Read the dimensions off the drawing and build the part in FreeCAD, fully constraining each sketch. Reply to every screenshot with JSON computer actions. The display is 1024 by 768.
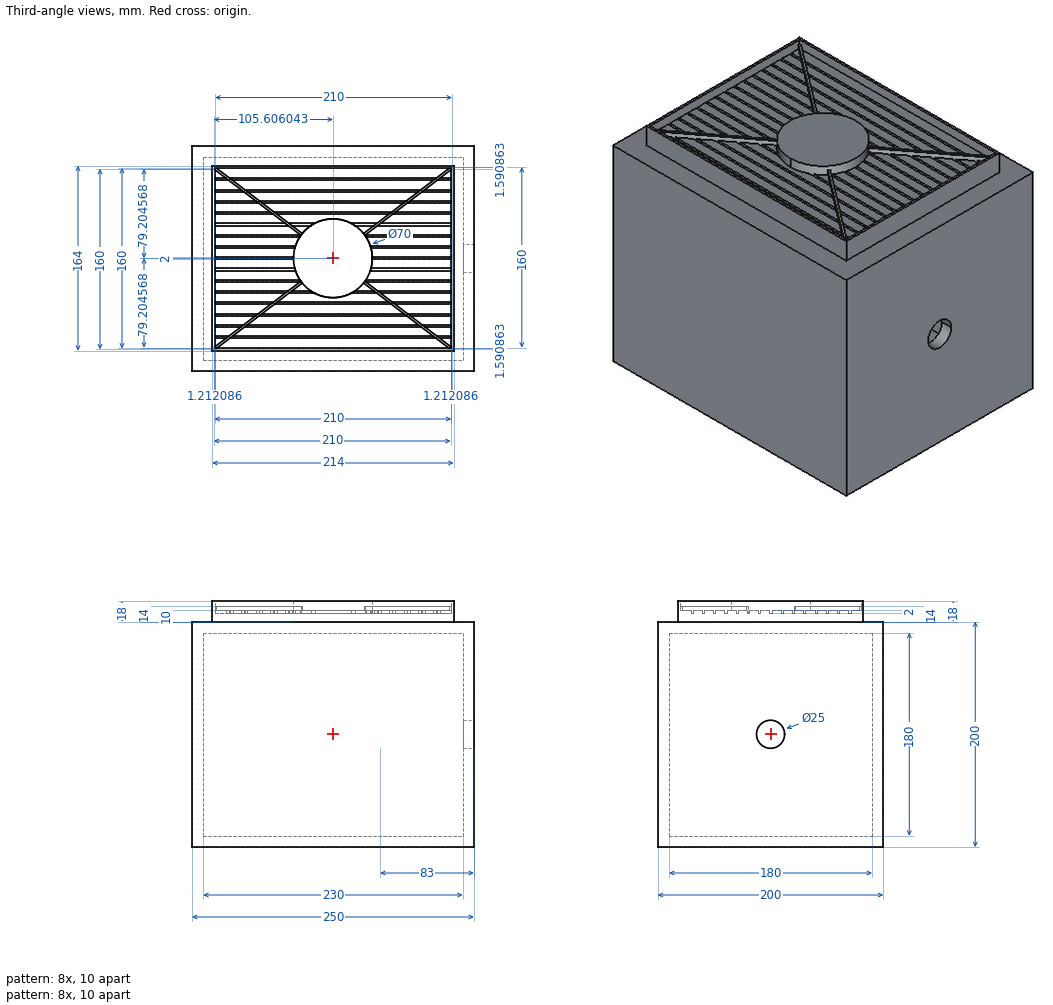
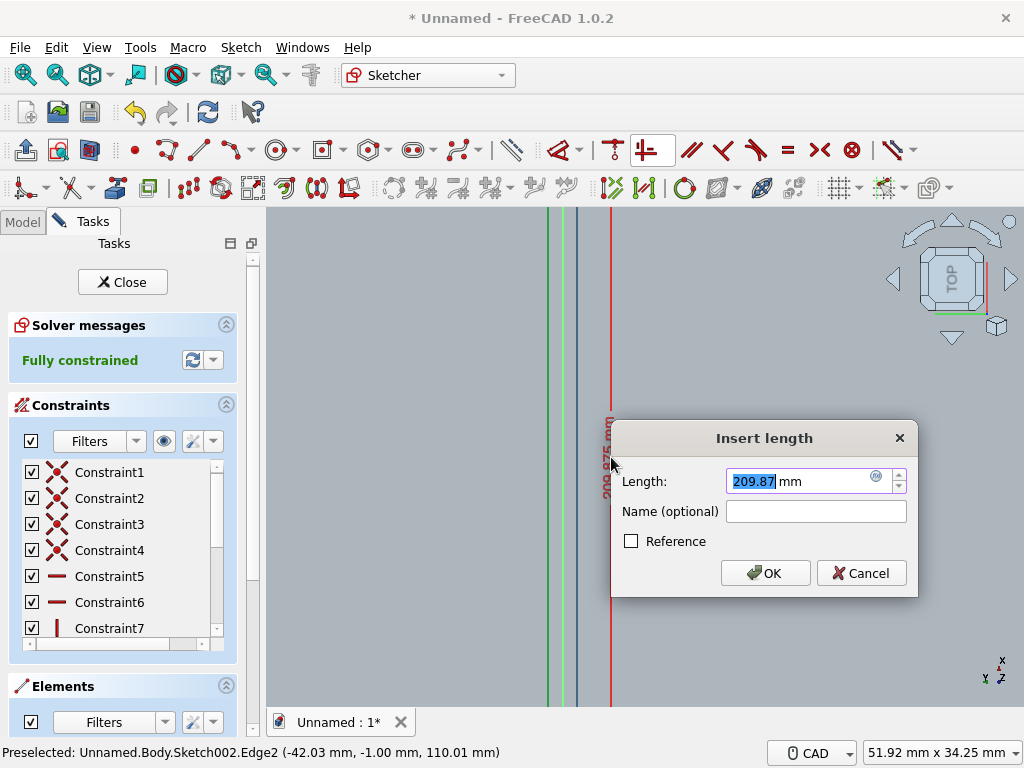
{"action": "type", "text": "210"}
{"action": "key", "text": "Return"}
{"action": "key", "text": "Escape"}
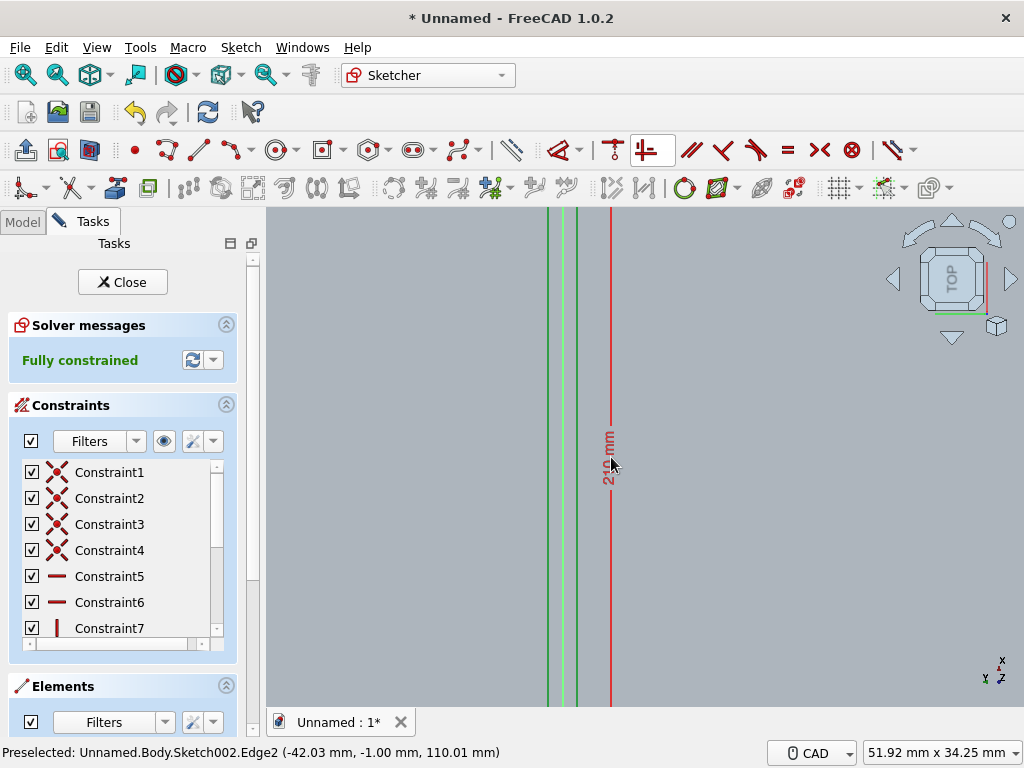
{"action": "left_click", "coordinate": [123, 282]}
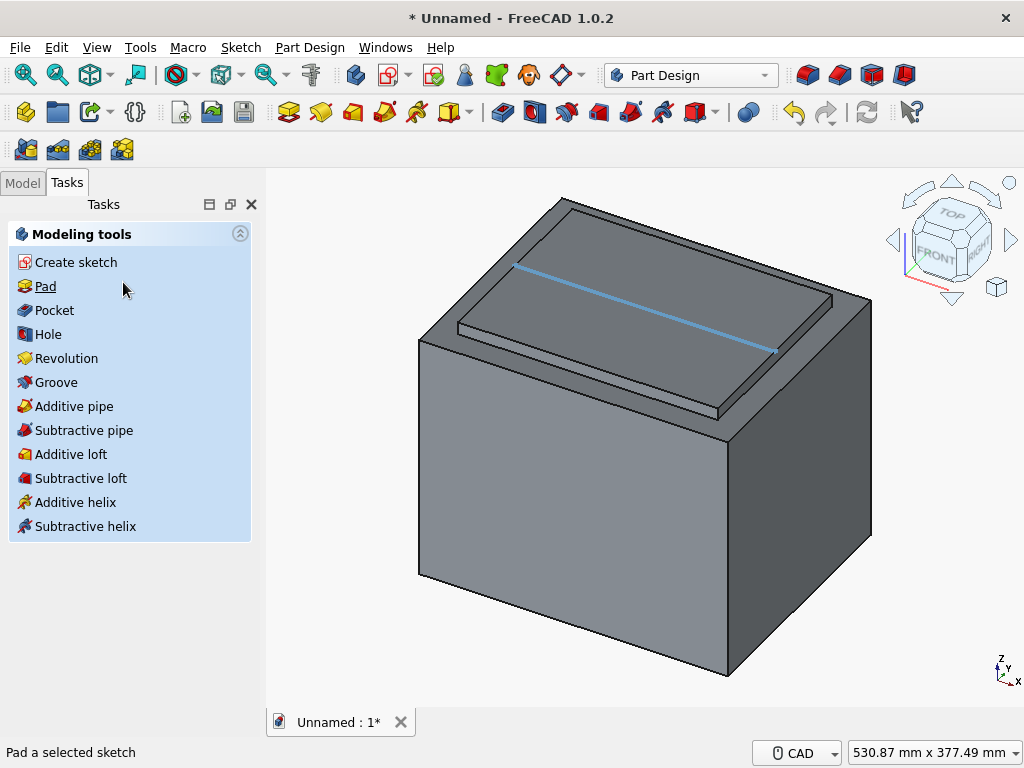
{"action": "left_click", "coordinate": [504, 112]}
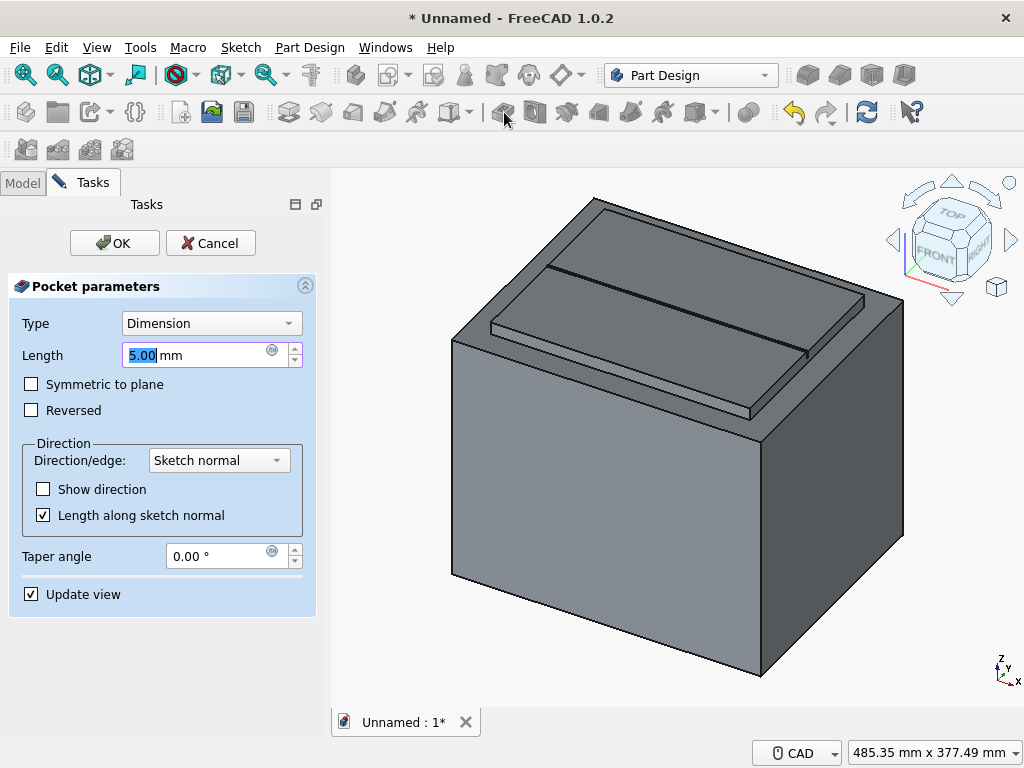
{"action": "type", "text": "2"}
{"action": "key", "text": "Tab"}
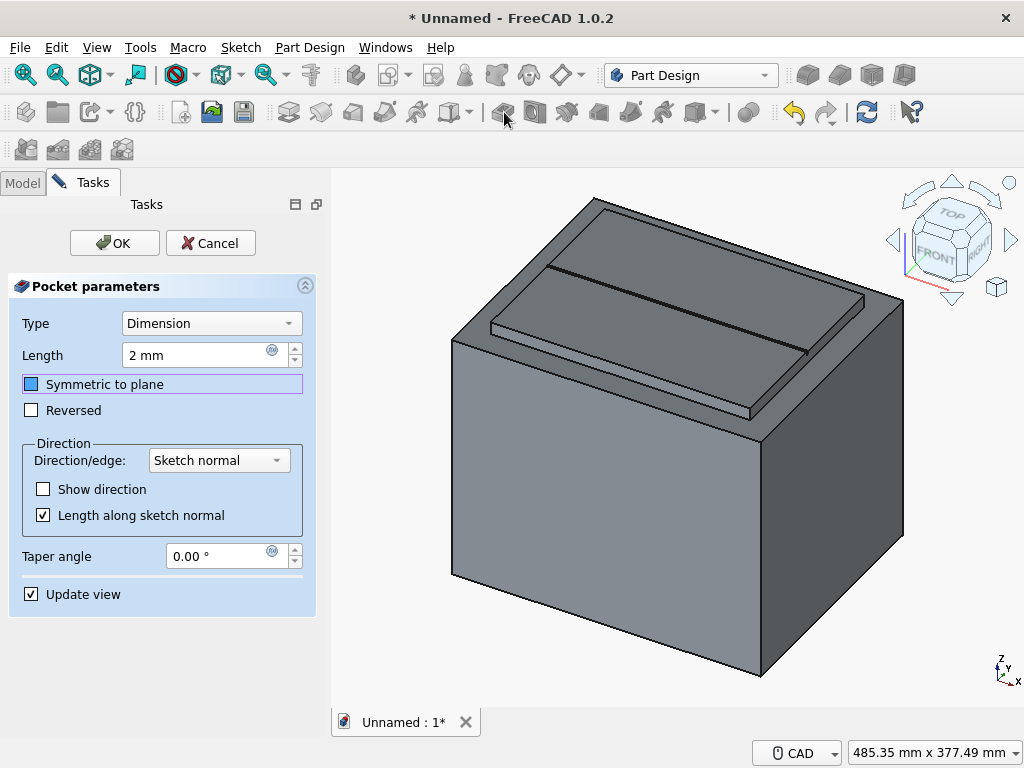
{"action": "left_click", "coordinate": [115, 243]}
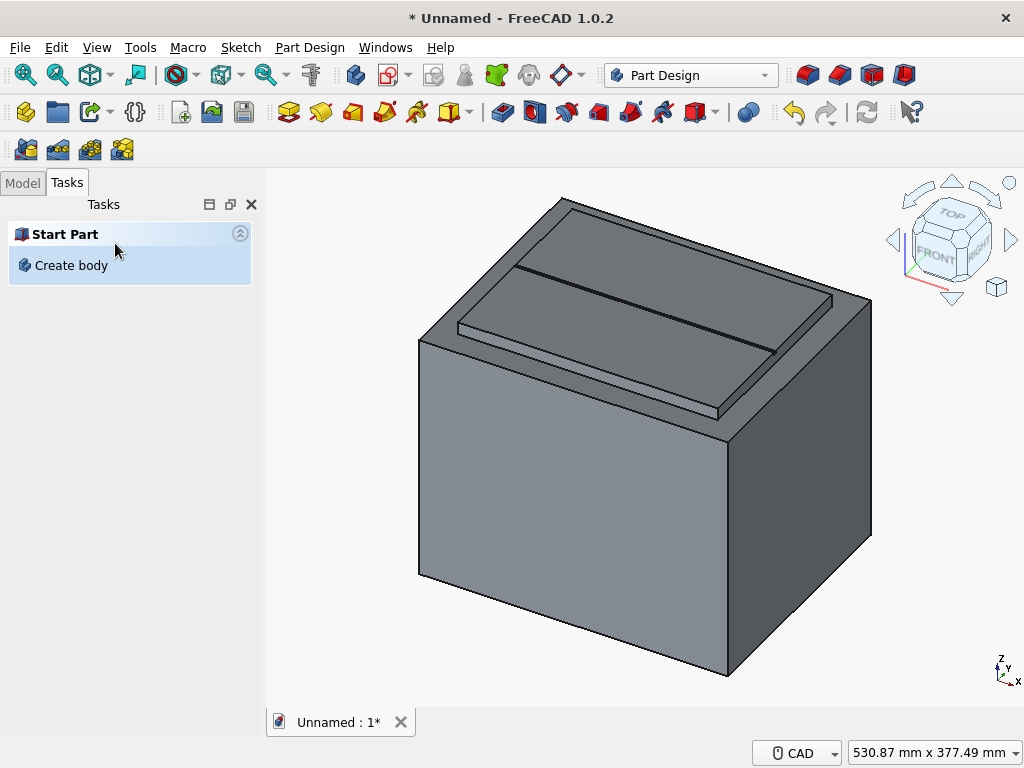
{"action": "left_click", "coordinate": [23, 182]}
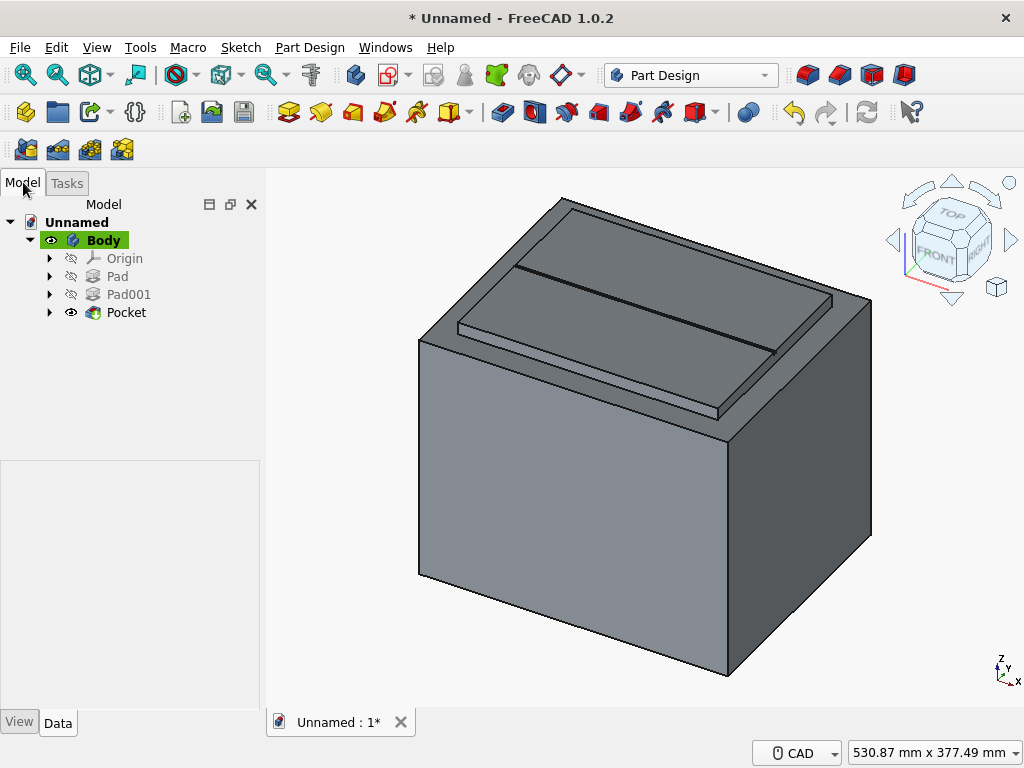
{"action": "left_click", "coordinate": [116, 312]}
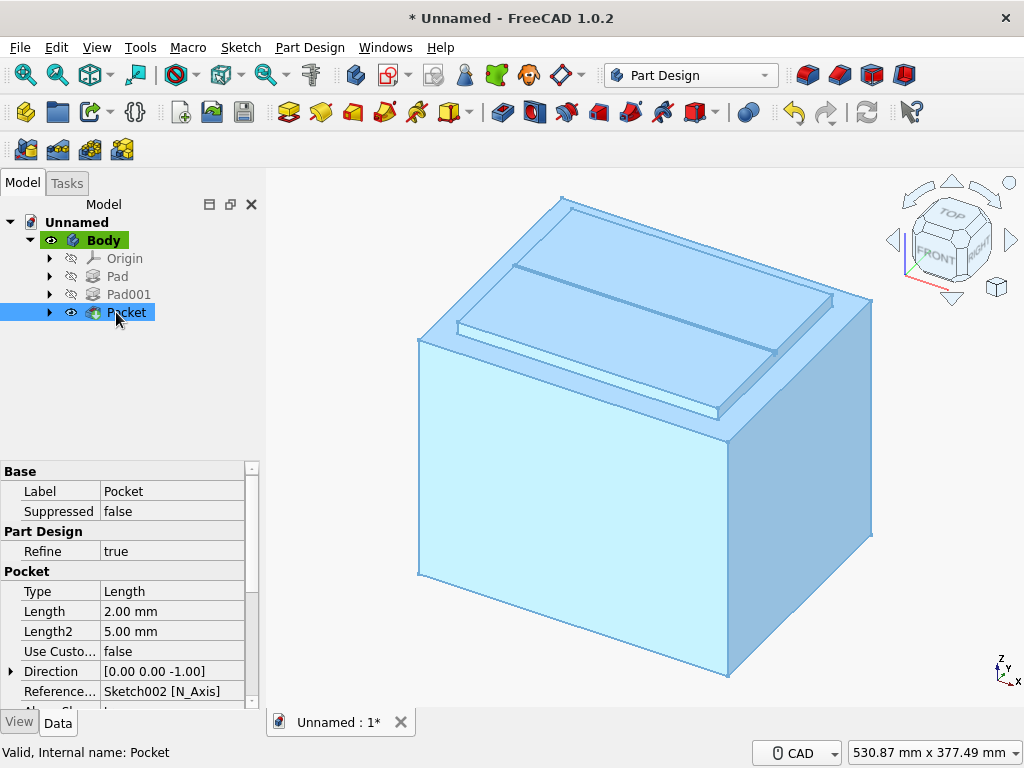
{"action": "left_click", "coordinate": [58, 150]}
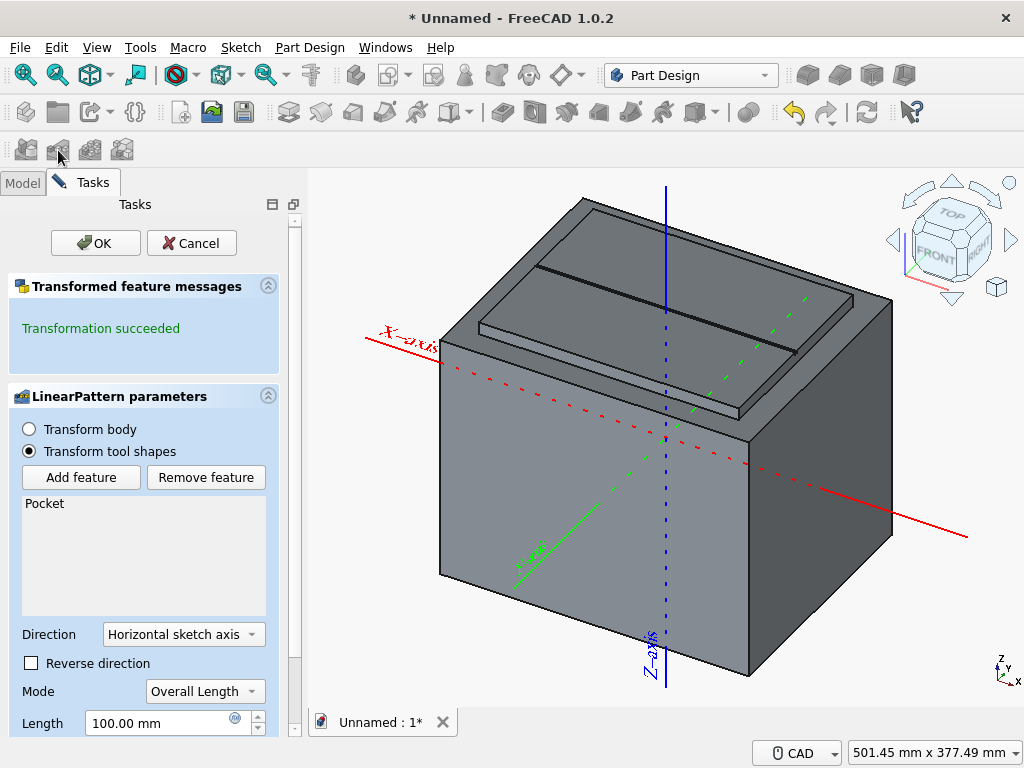
{"action": "left_click", "coordinate": [184, 634]}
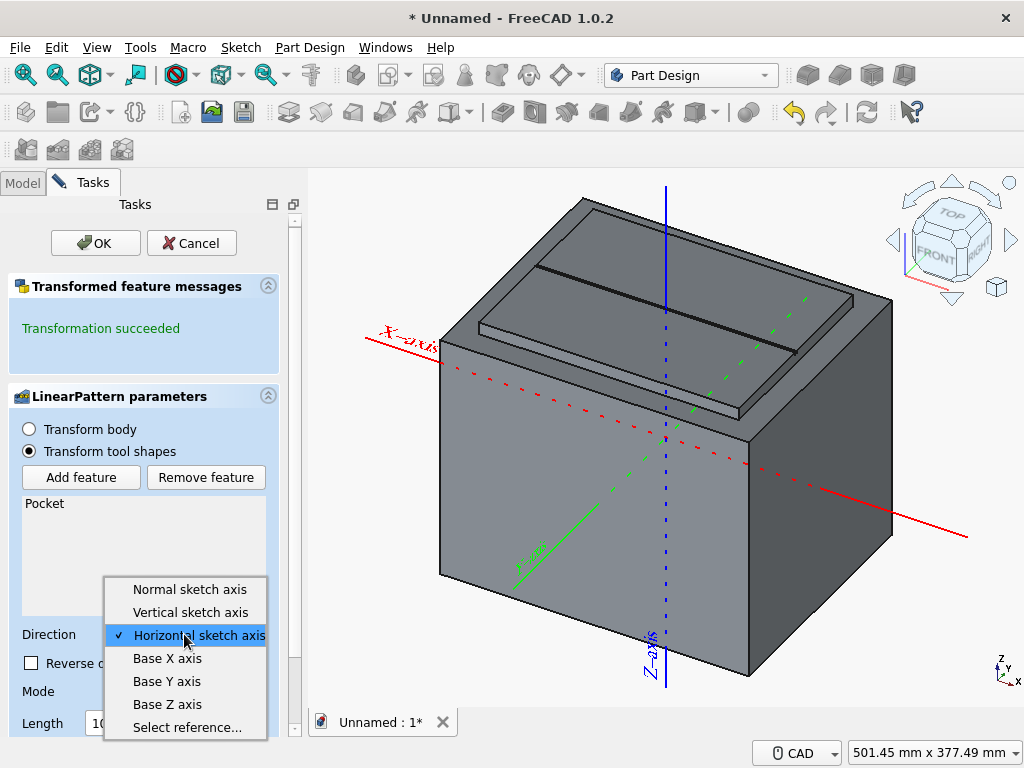
{"action": "left_click", "coordinate": [184, 682]}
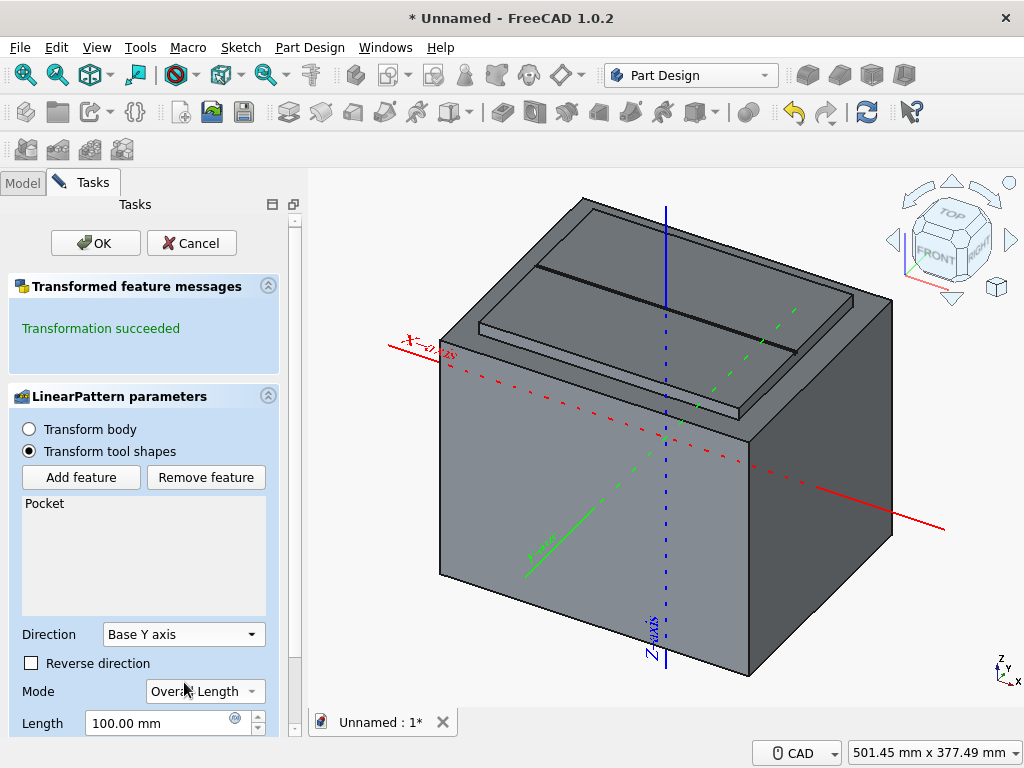
{"action": "left_click", "coordinate": [206, 692]}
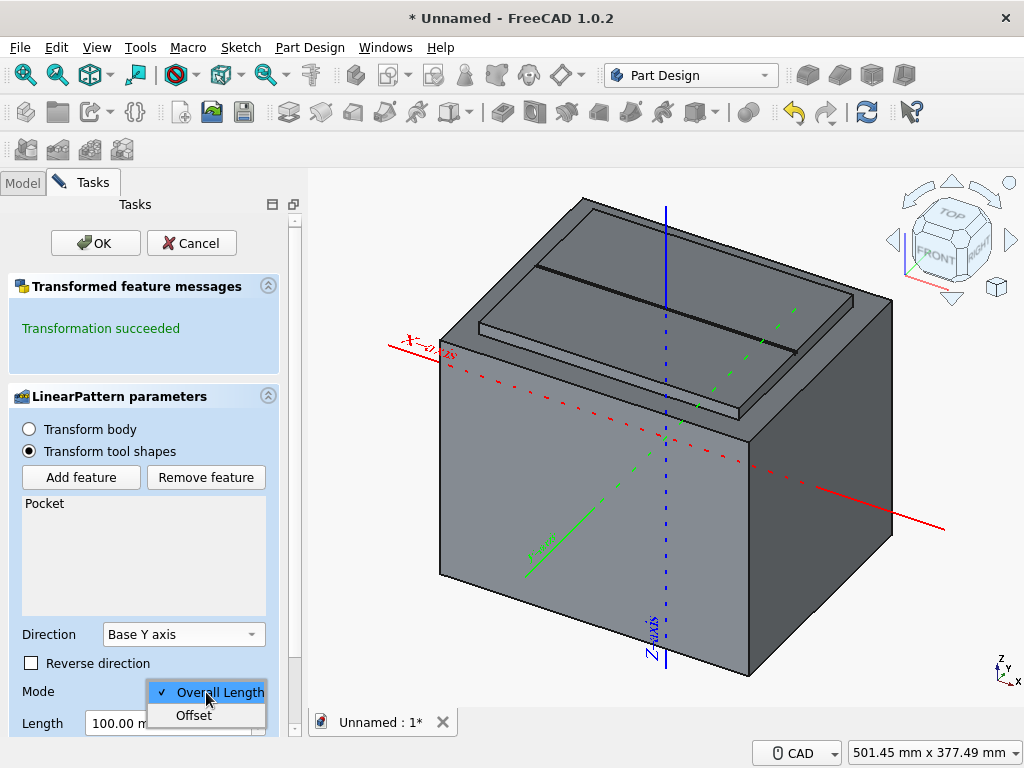
{"action": "left_click", "coordinate": [206, 716]}